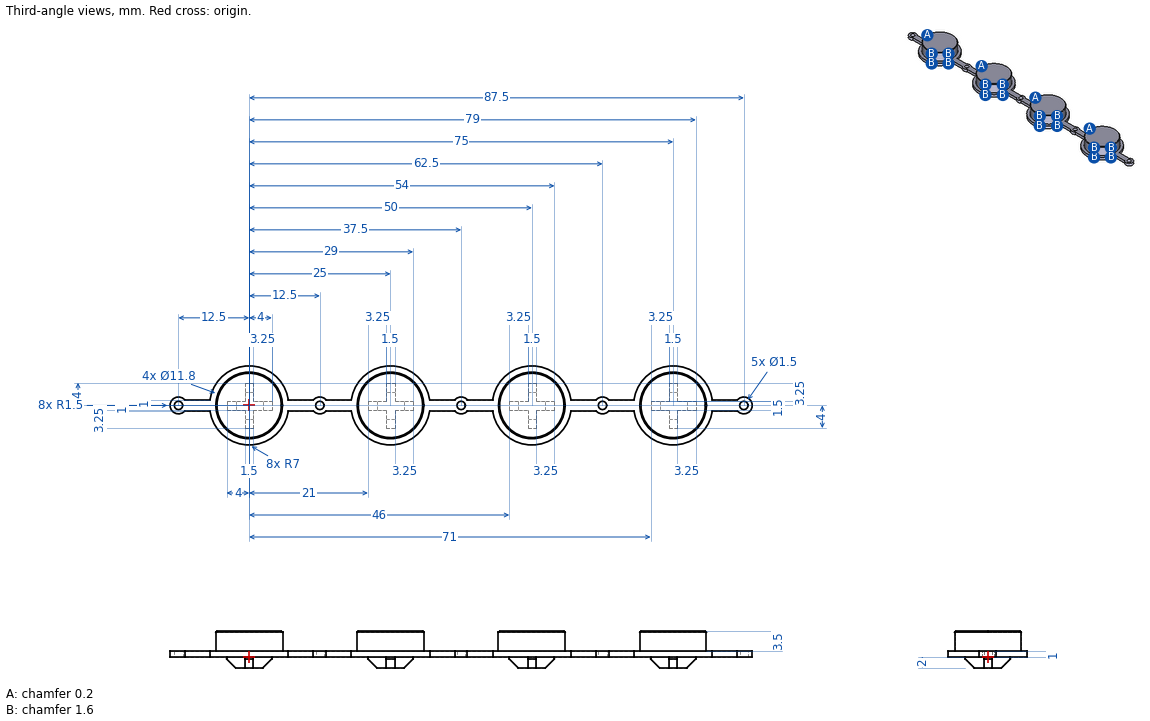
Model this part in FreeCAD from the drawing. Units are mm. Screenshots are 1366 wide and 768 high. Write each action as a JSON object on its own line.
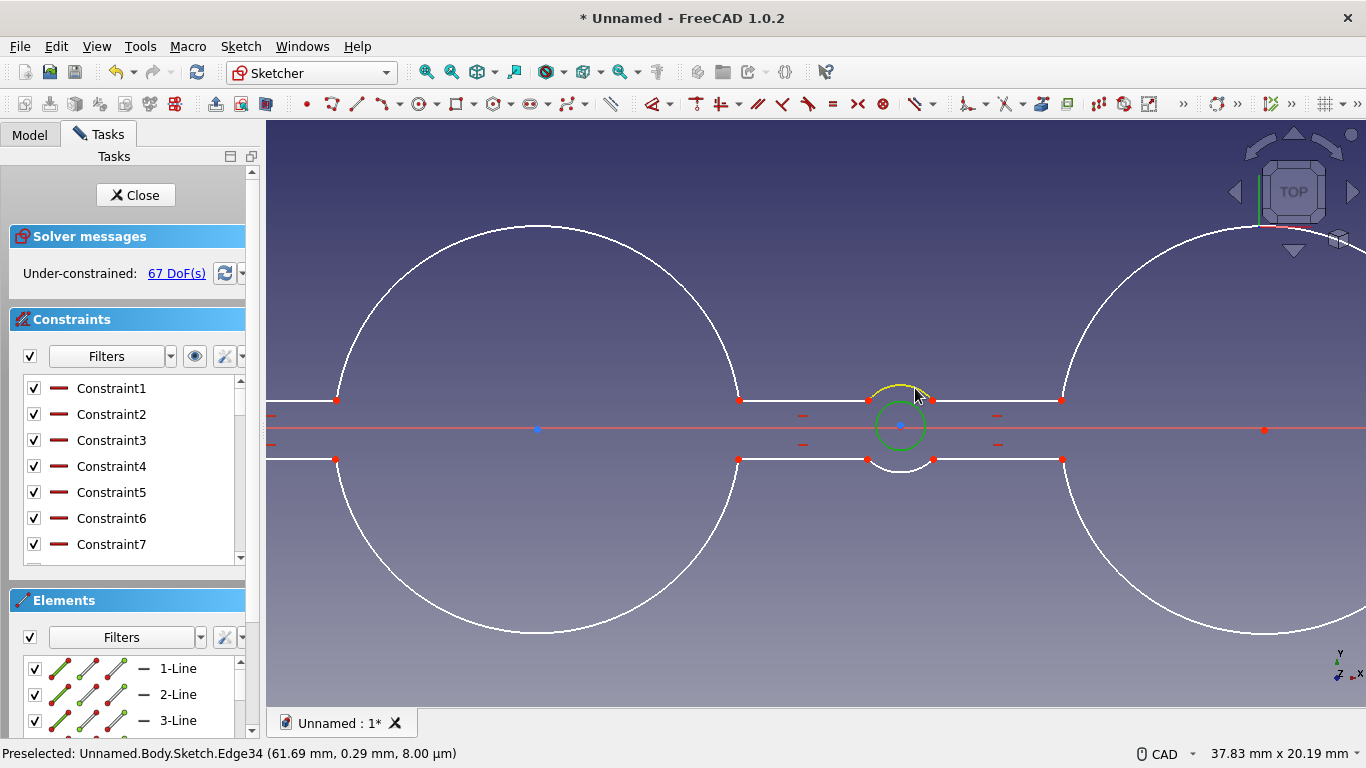
{"action": "left_click", "coordinate": [915, 388]}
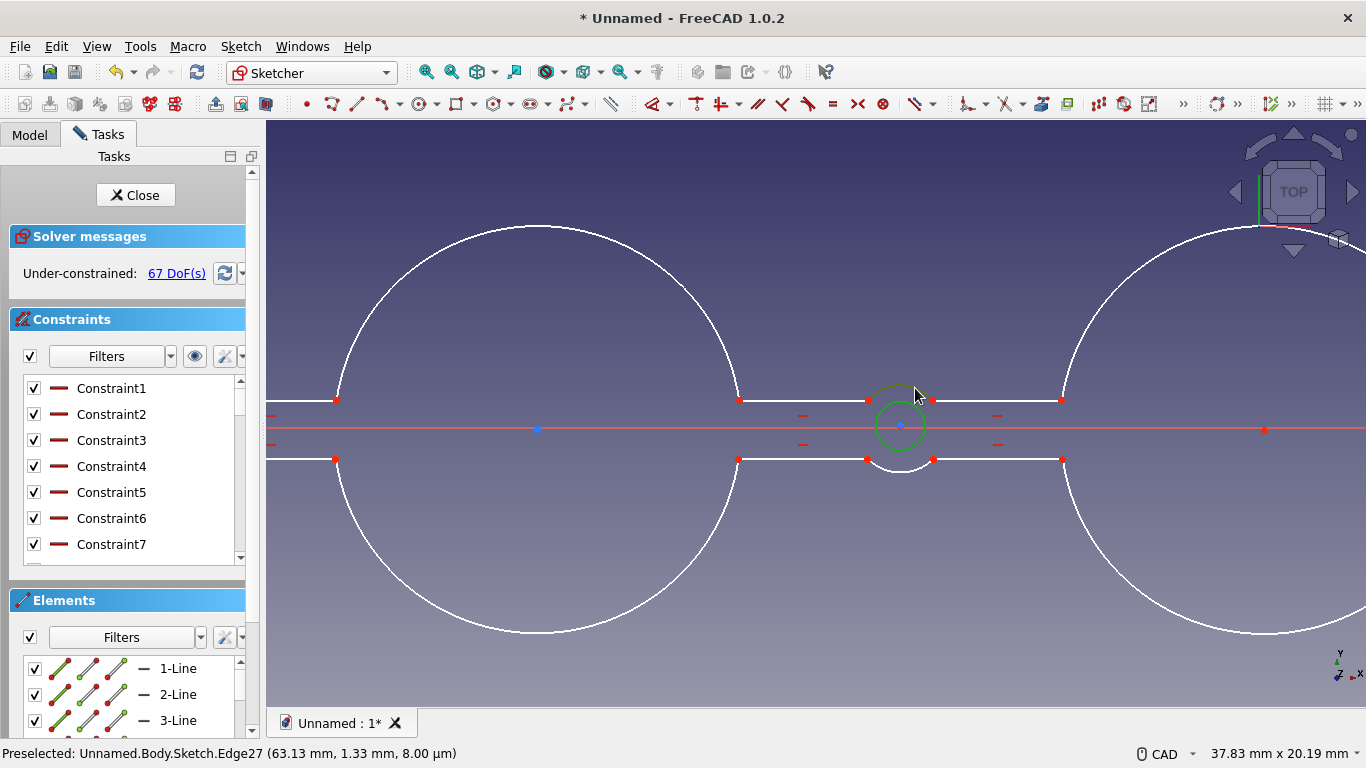
{"action": "key", "text": "c"}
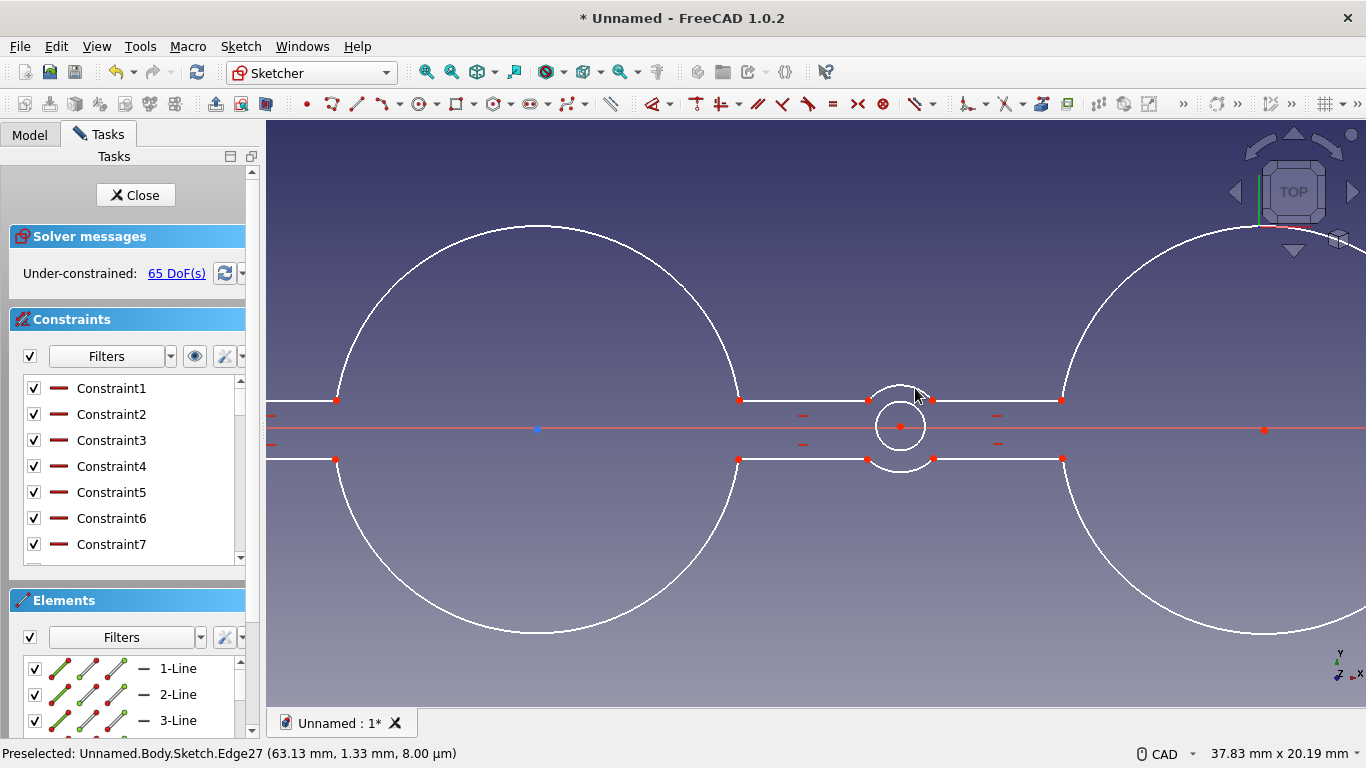
{"action": "scroll", "coordinate": [893, 410], "scroll_direction": "down", "scroll_amount": 8}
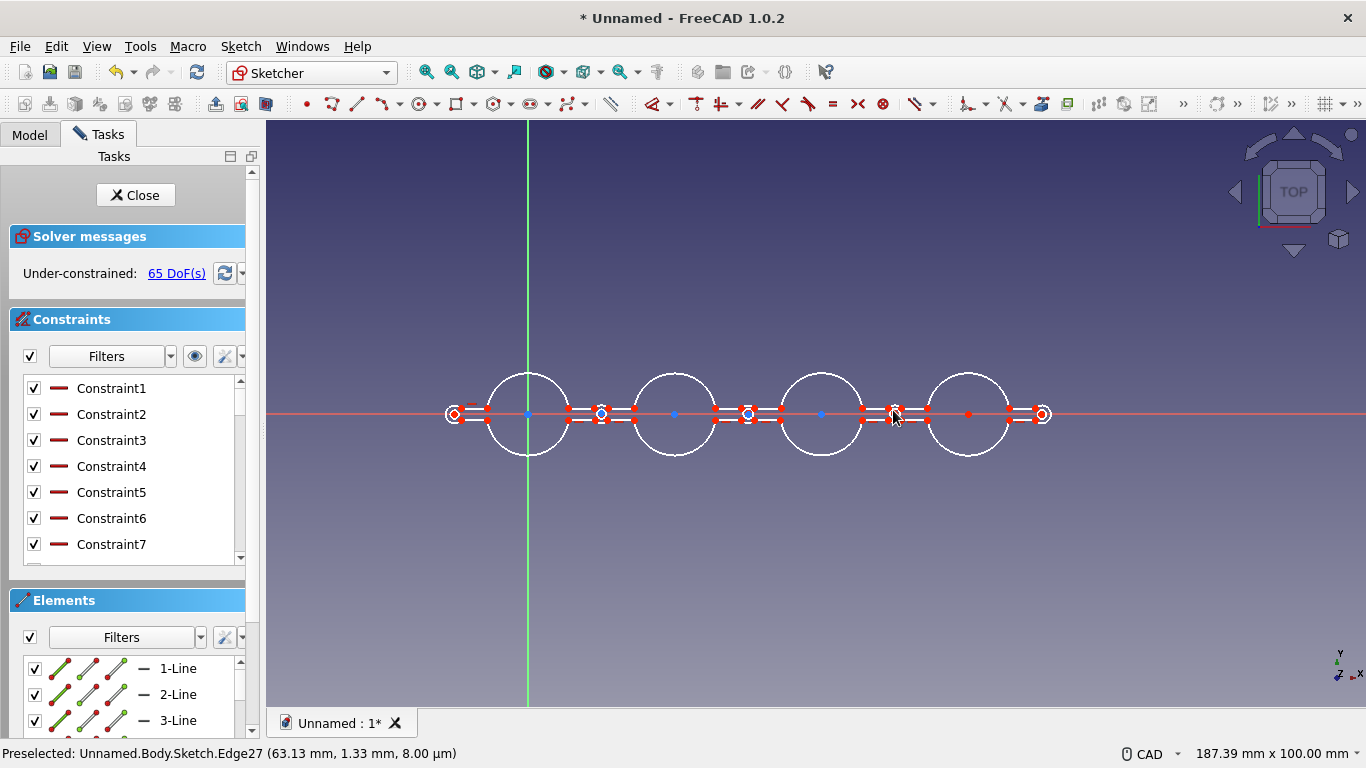
{"action": "left_click", "coordinate": [799, 449]}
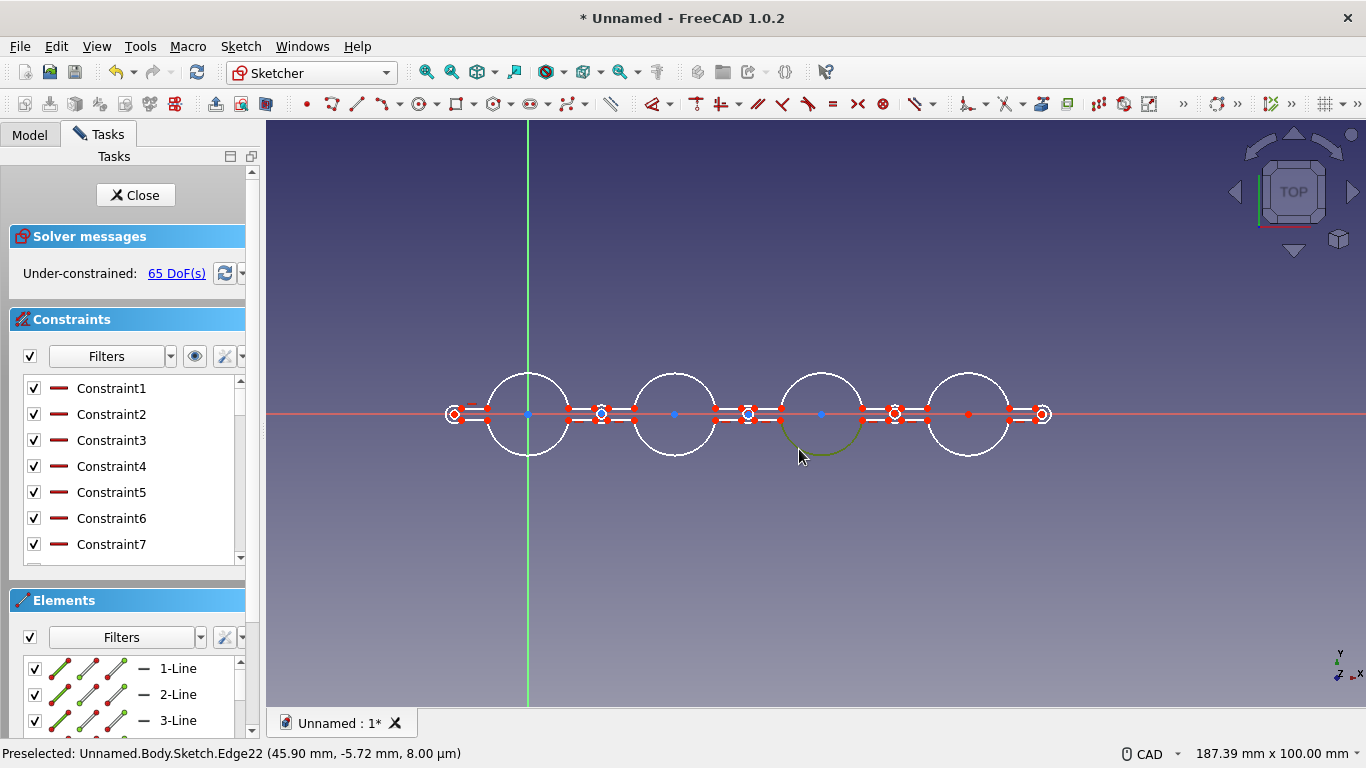
{"action": "left_click", "coordinate": [844, 380]}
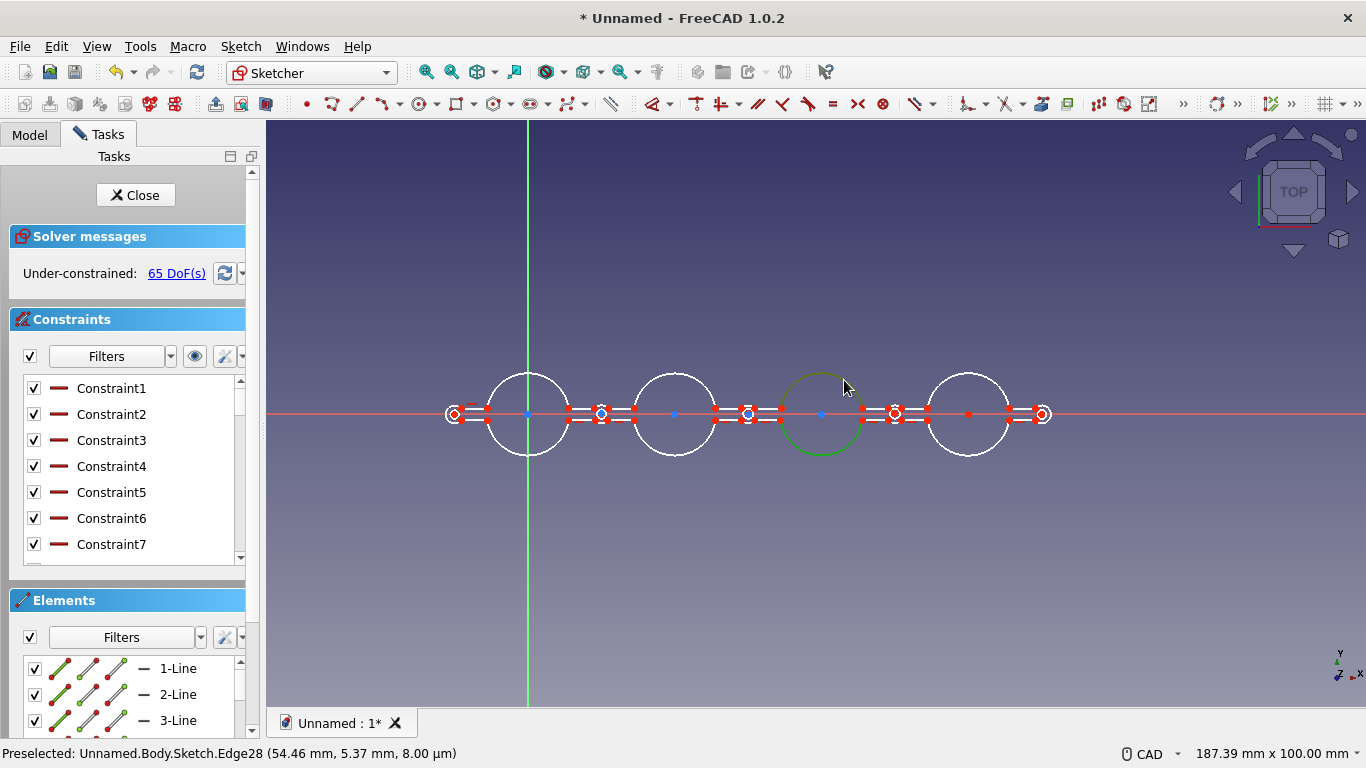
{"action": "key", "text": "c"}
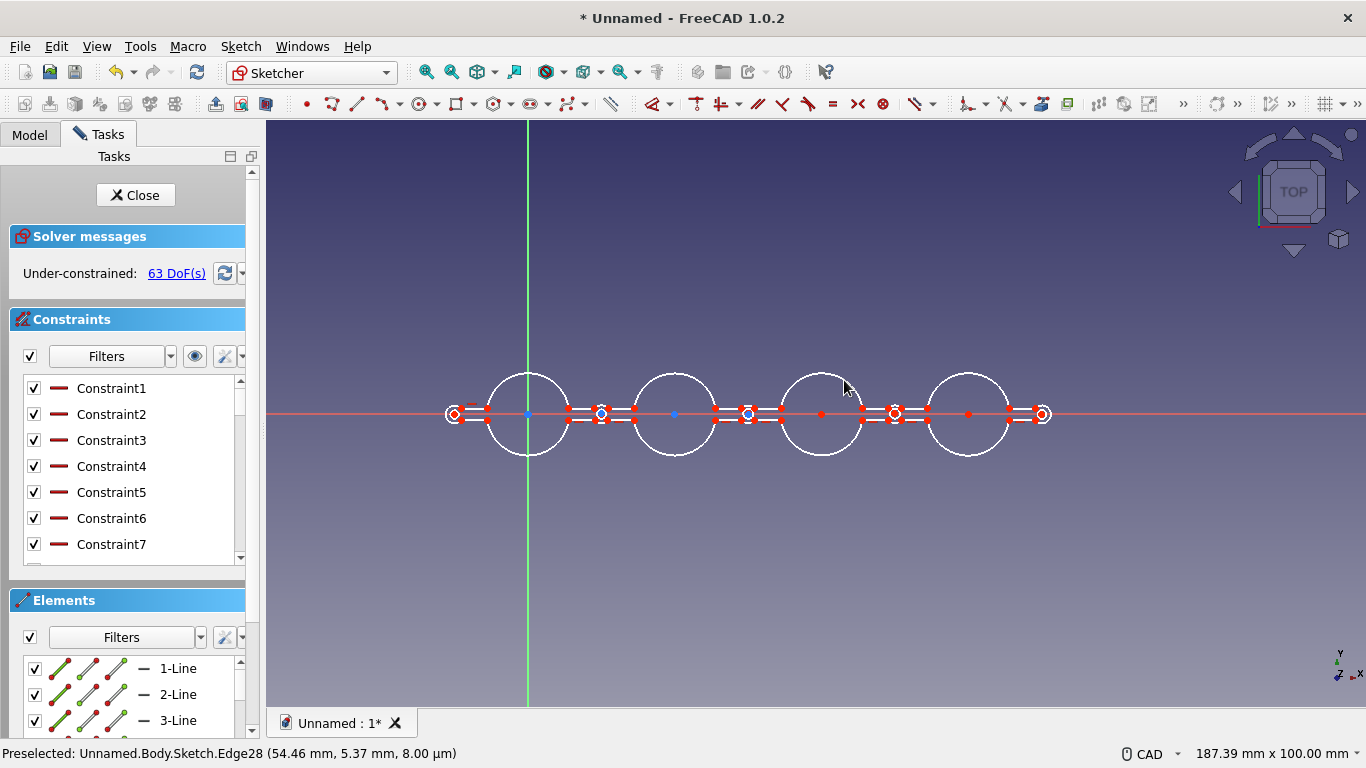
{"action": "scroll", "coordinate": [743, 414], "scroll_direction": "up", "scroll_amount": 6}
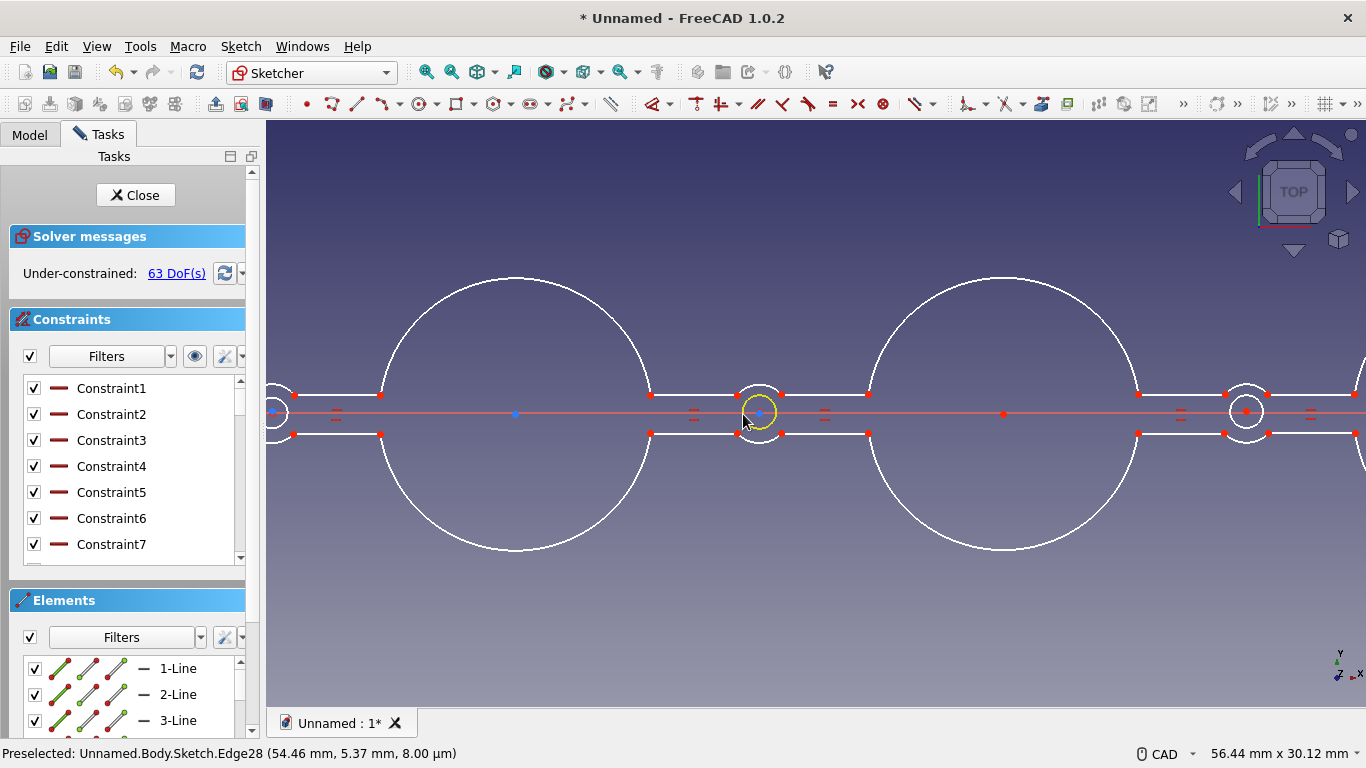
{"action": "left_click", "coordinate": [743, 412]}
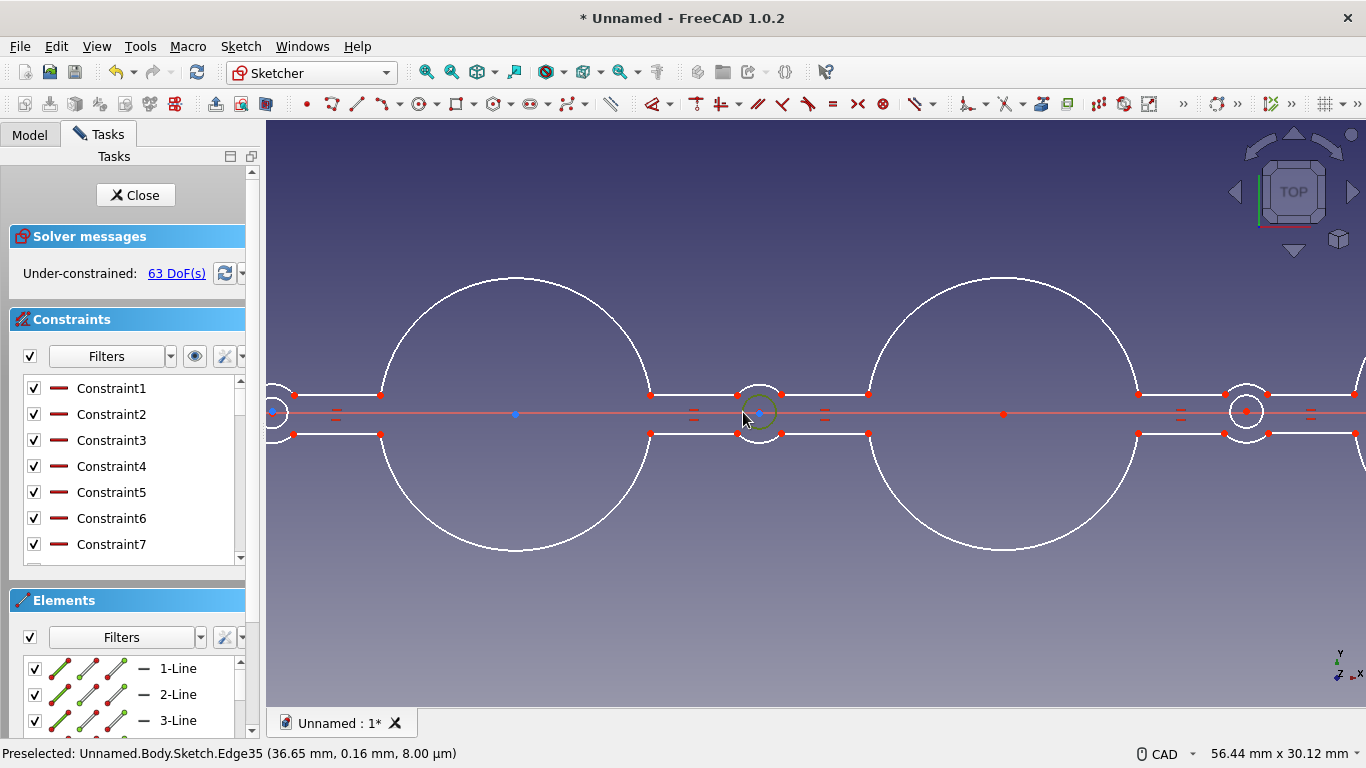
{"action": "scroll", "coordinate": [769, 386], "scroll_direction": "up", "scroll_amount": 2}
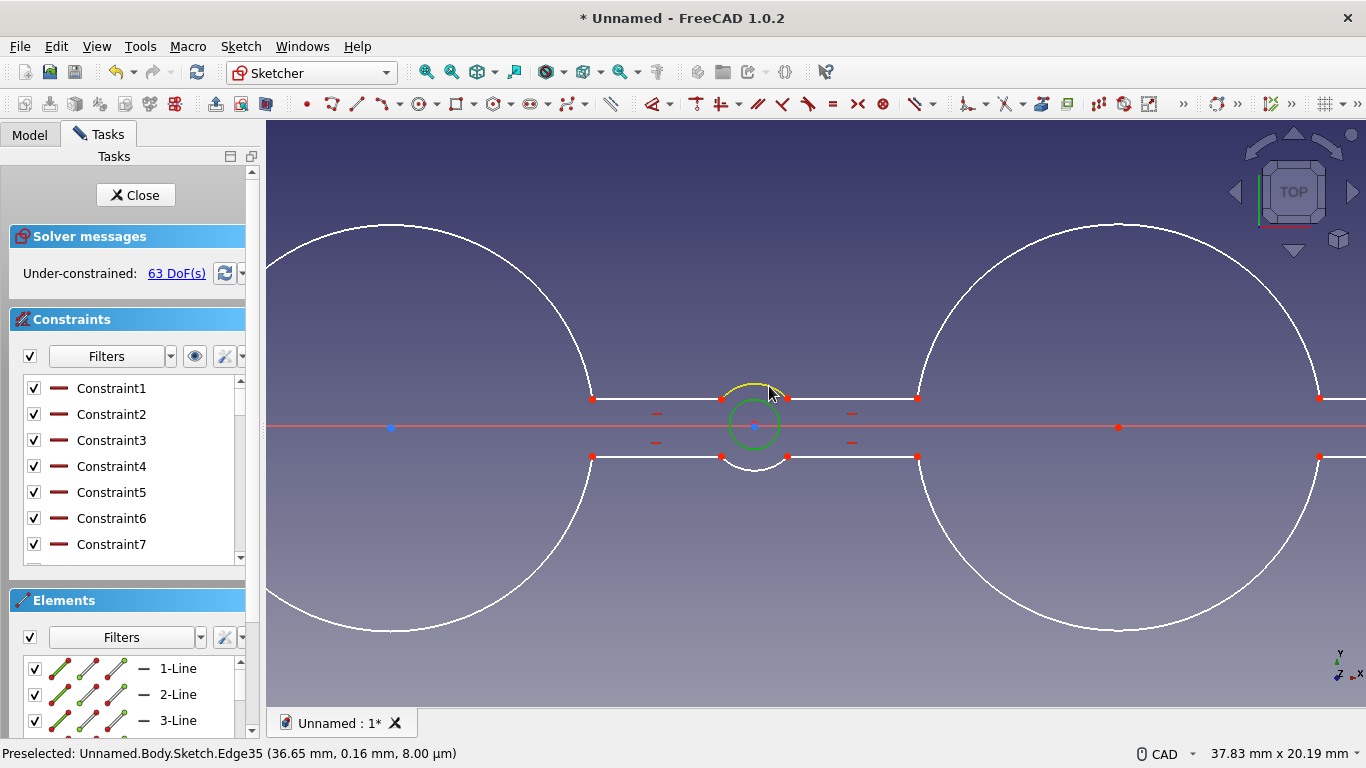
{"action": "left_click", "coordinate": [769, 386]}